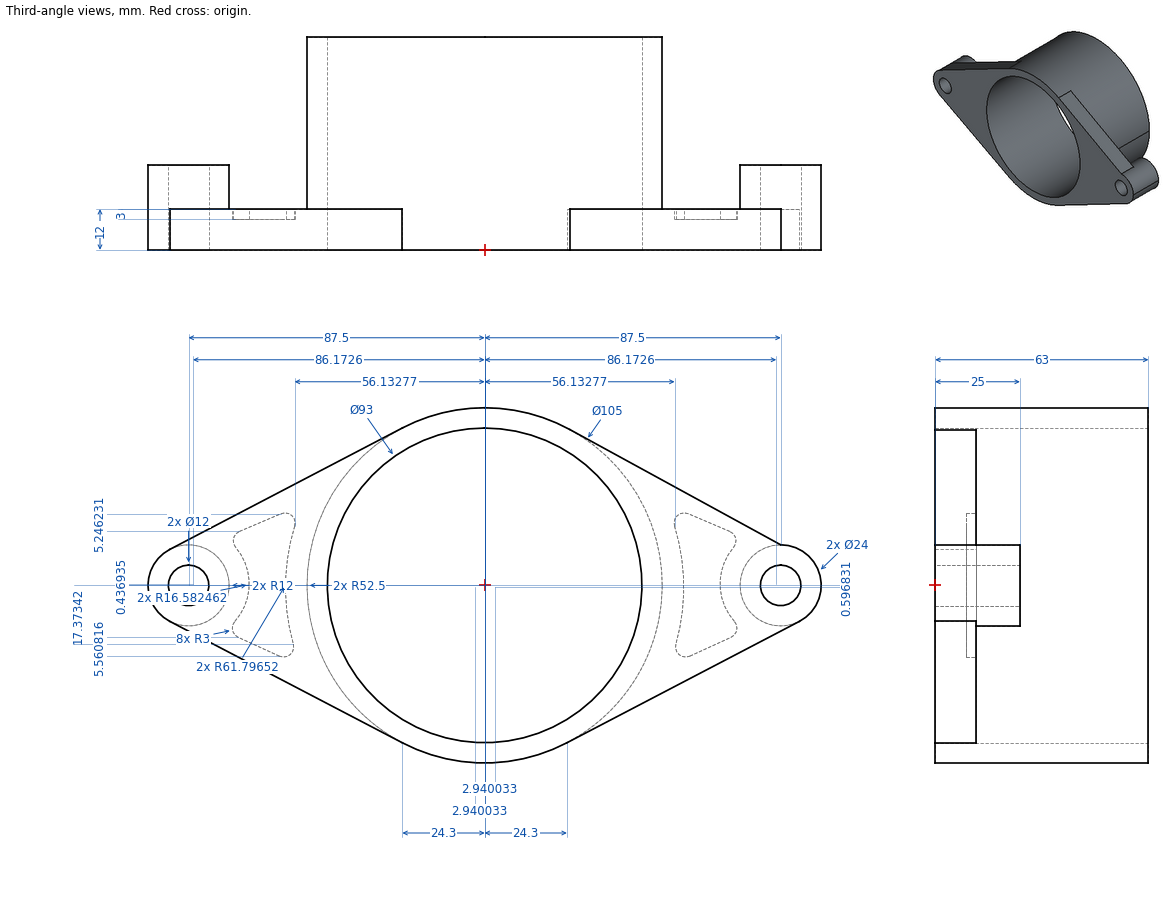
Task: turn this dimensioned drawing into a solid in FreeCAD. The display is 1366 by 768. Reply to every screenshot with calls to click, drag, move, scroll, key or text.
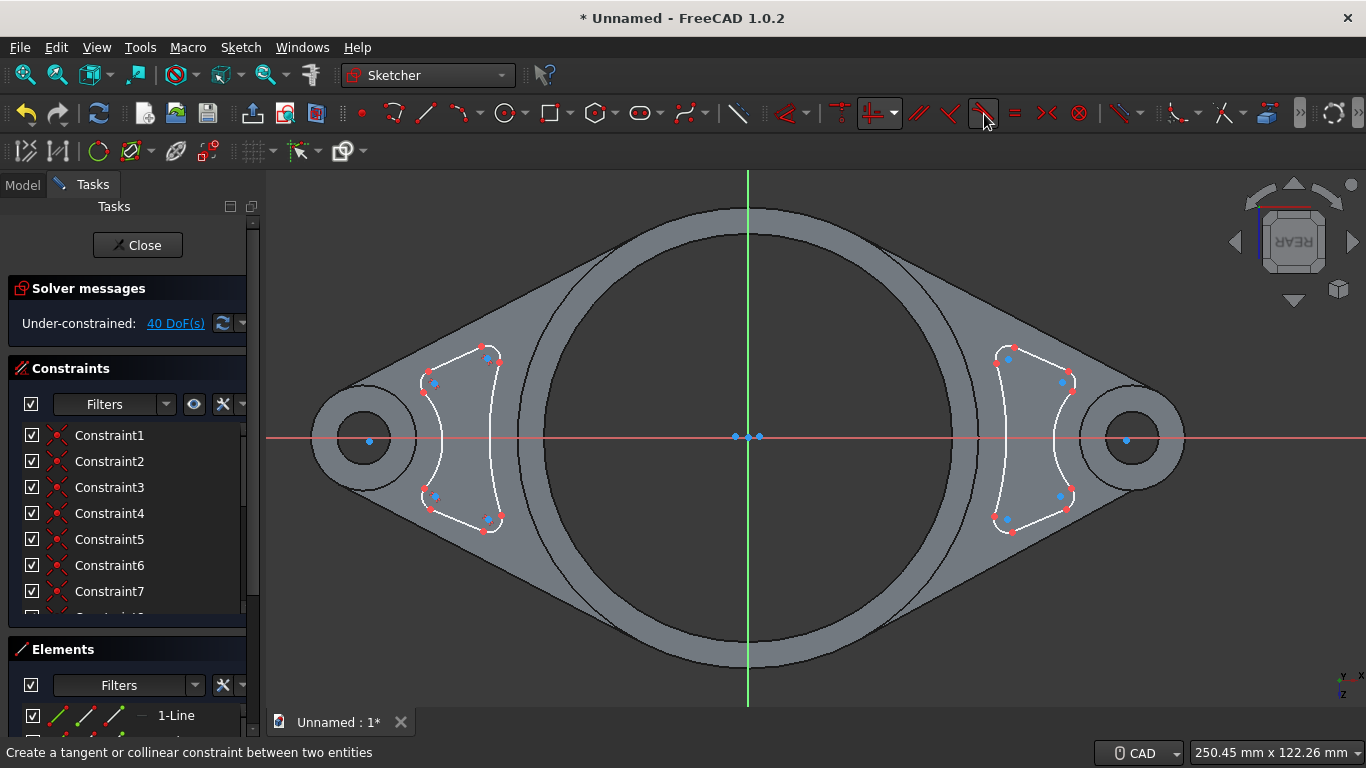
click(421, 381)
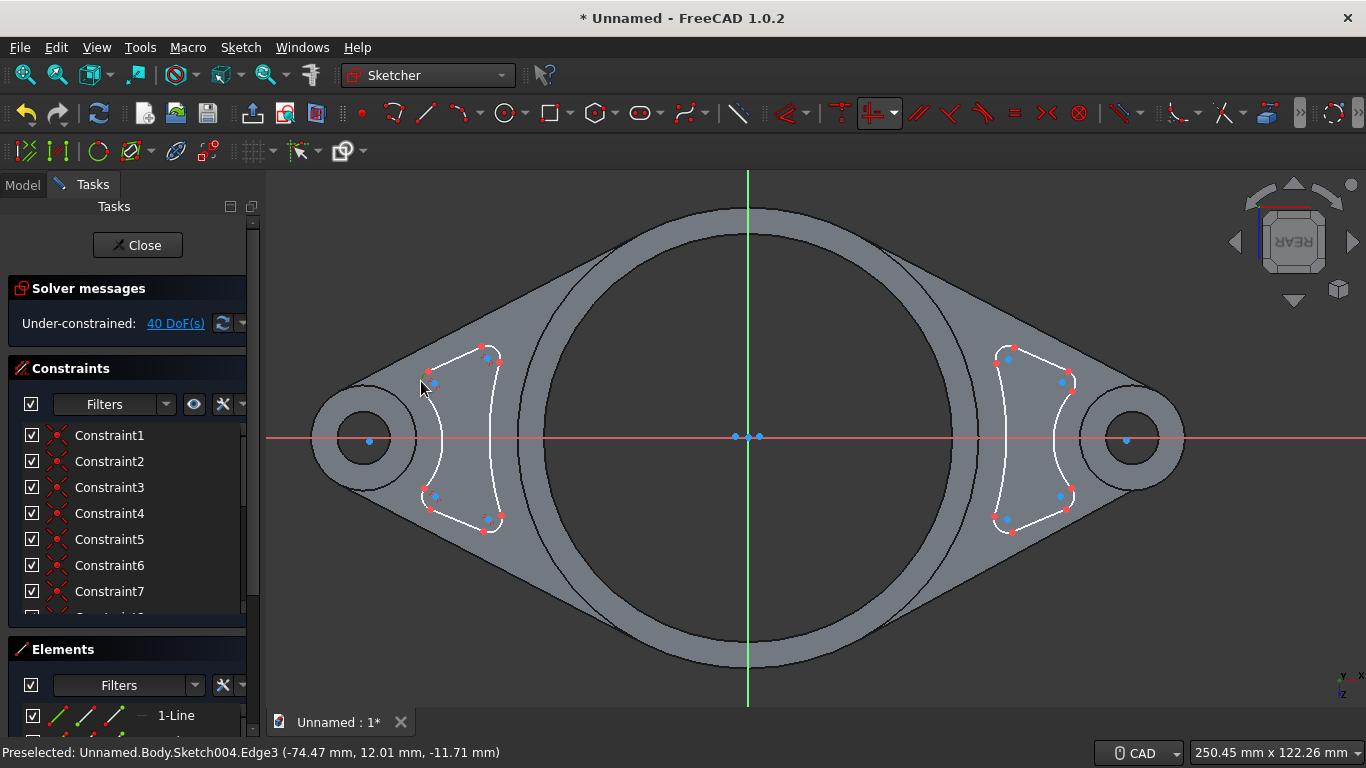
click(440, 461)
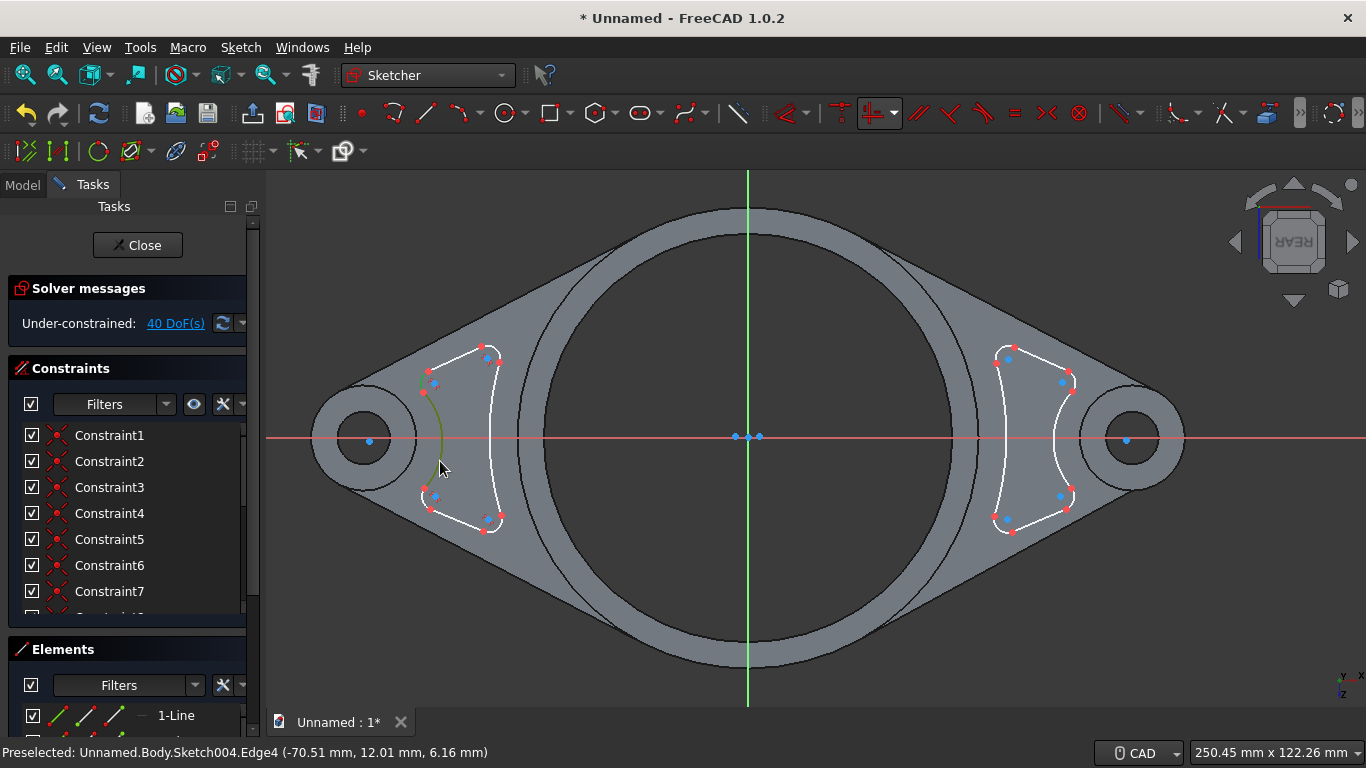
key(t)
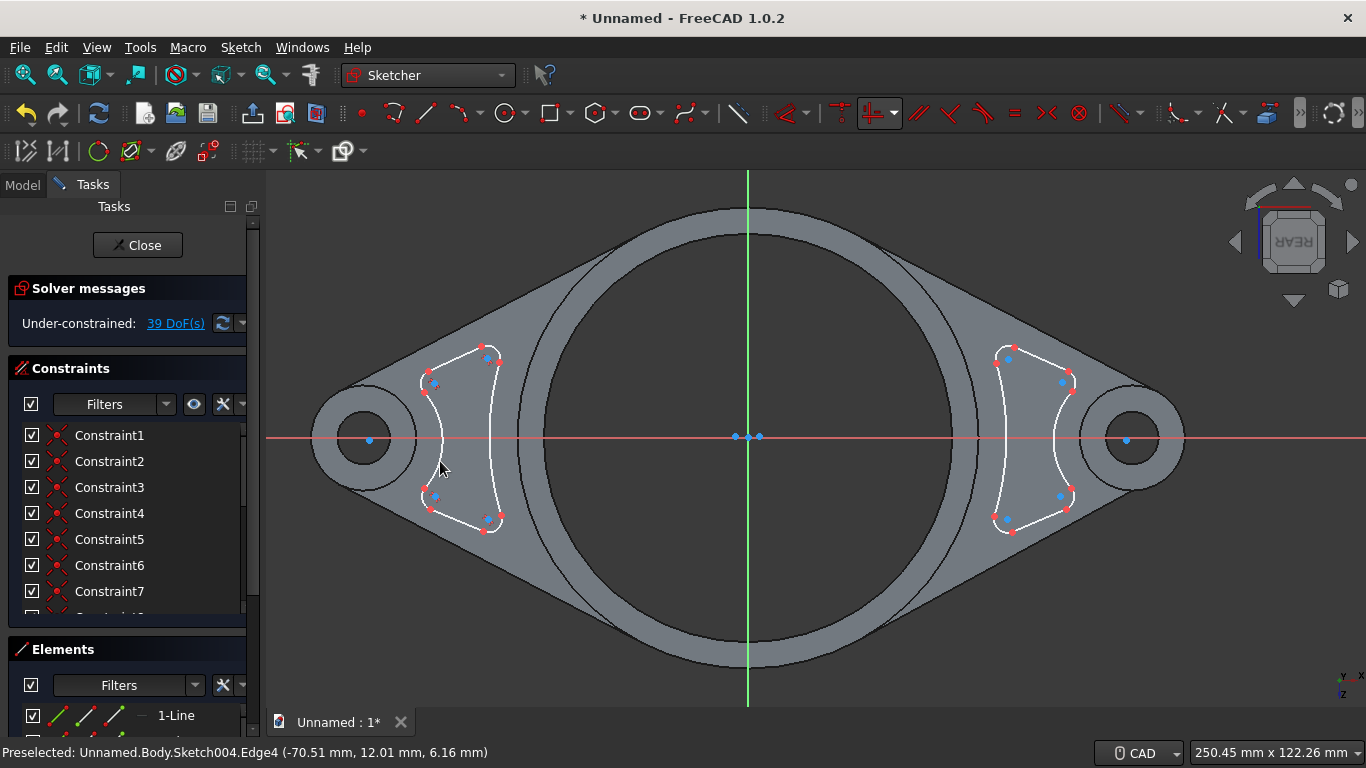
click(440, 461)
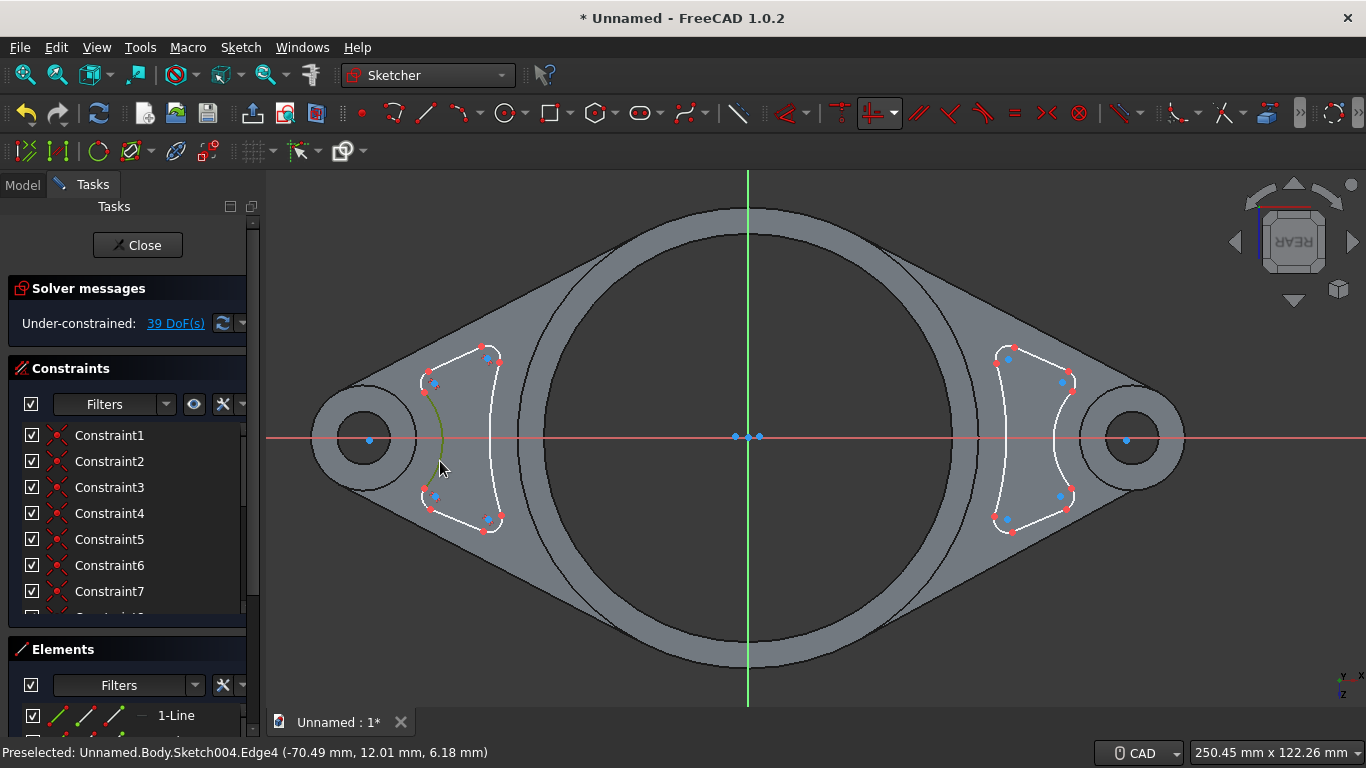
click(423, 500)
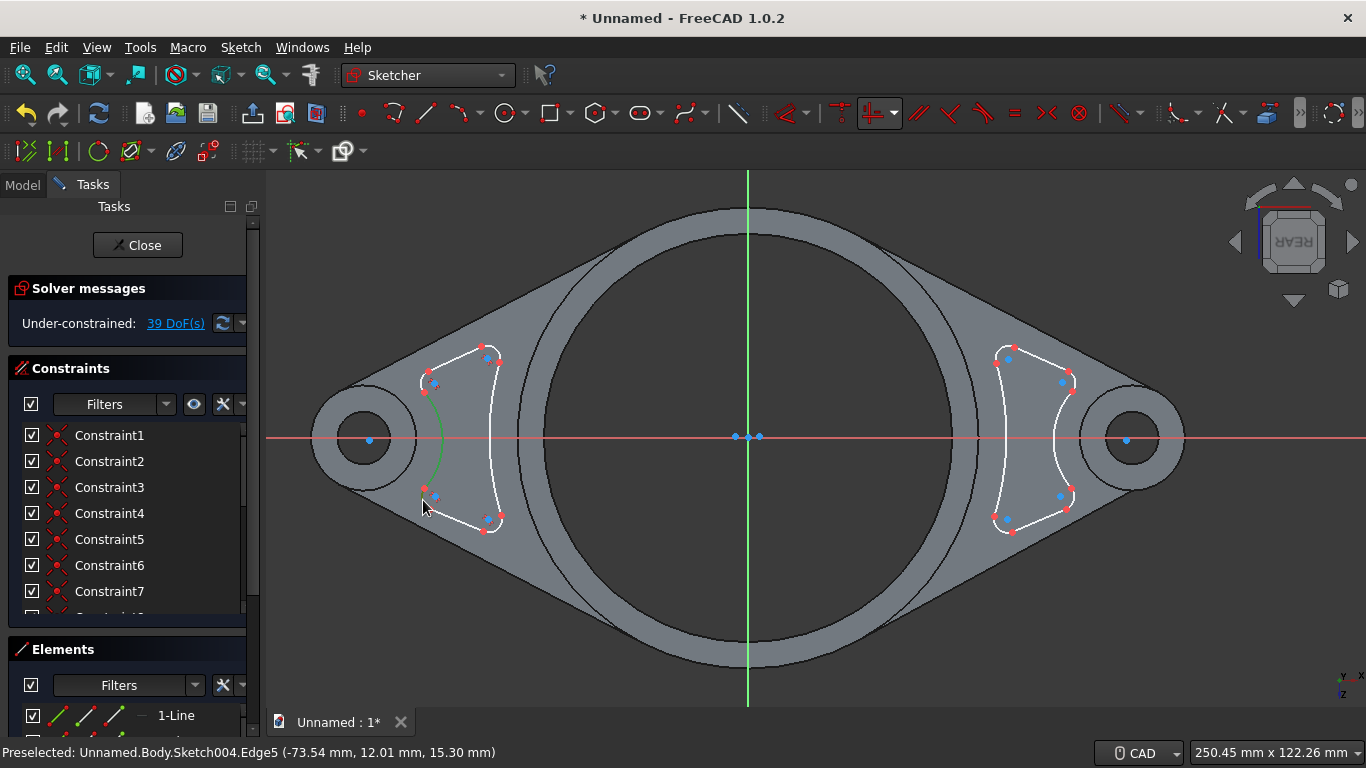
click(984, 114)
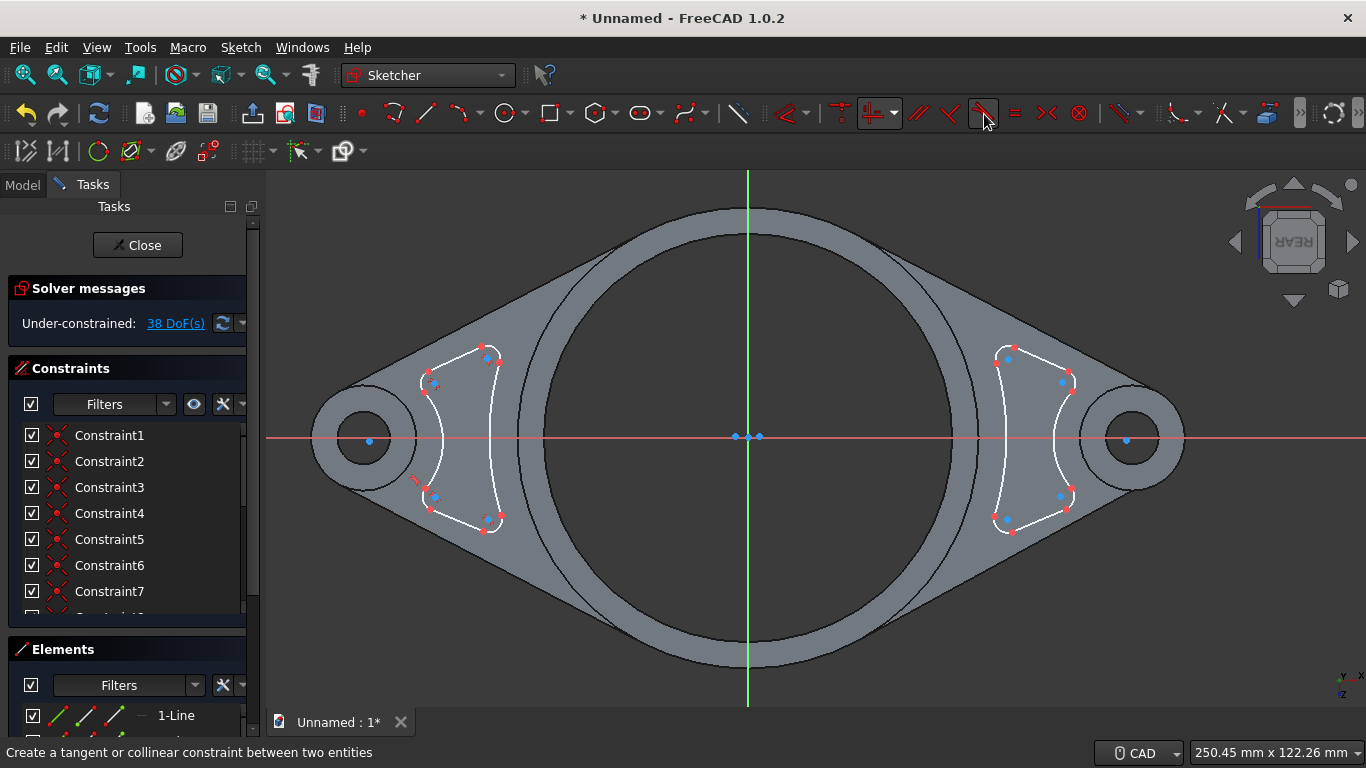
click(498, 529)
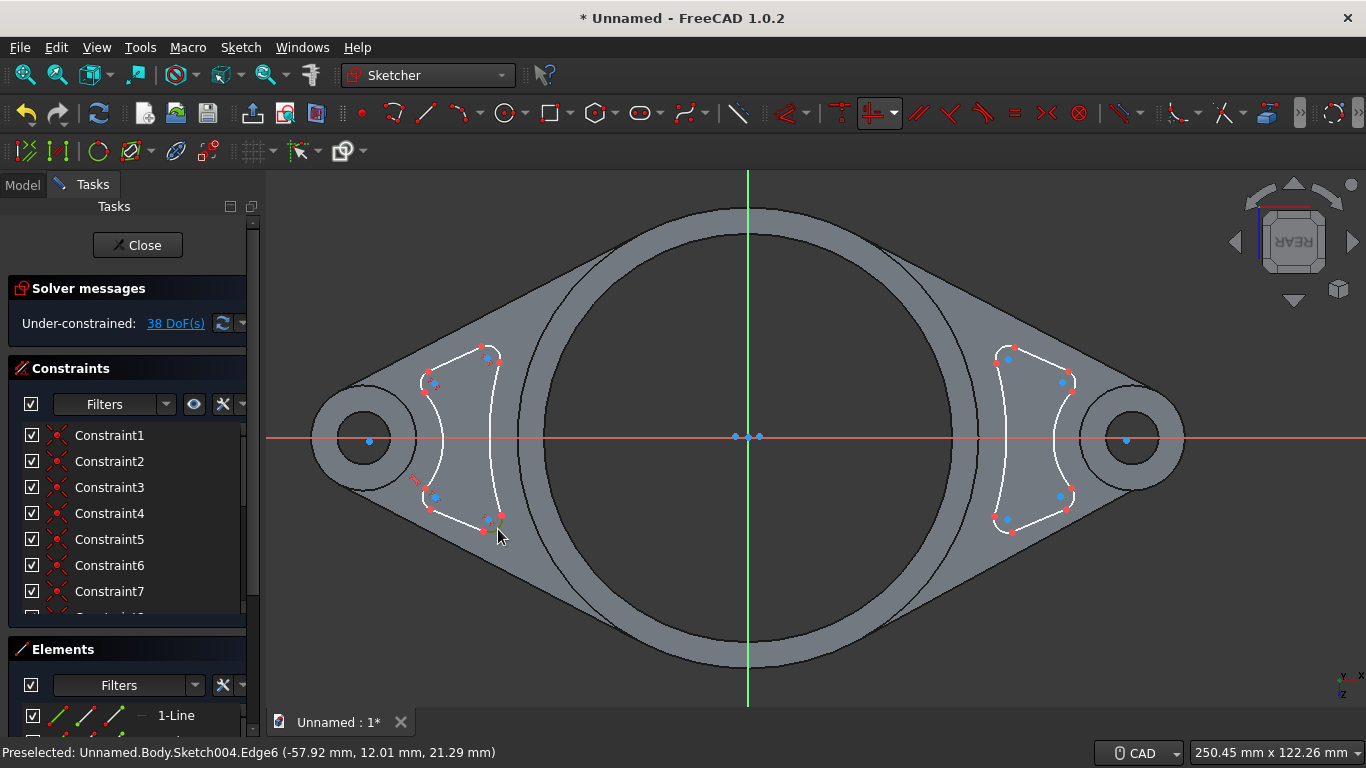
click(491, 408)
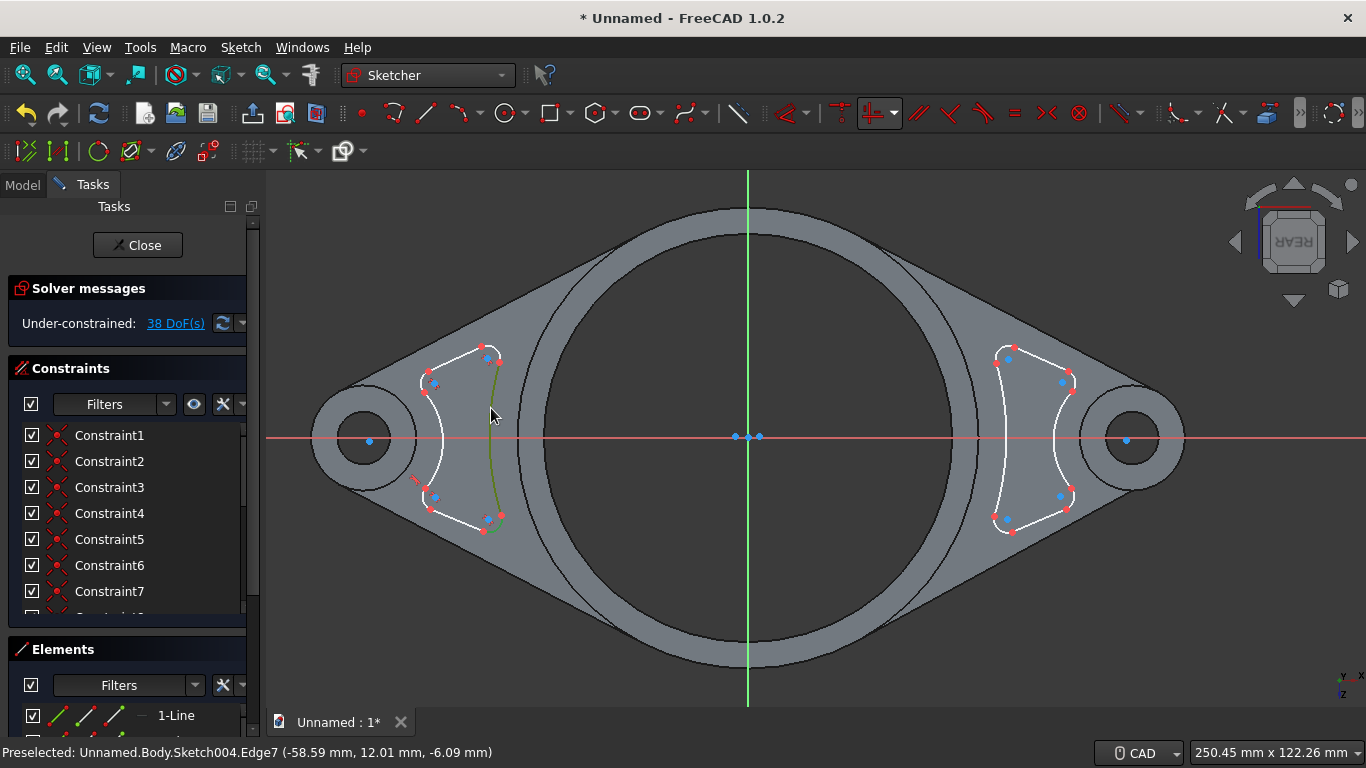
key(t)